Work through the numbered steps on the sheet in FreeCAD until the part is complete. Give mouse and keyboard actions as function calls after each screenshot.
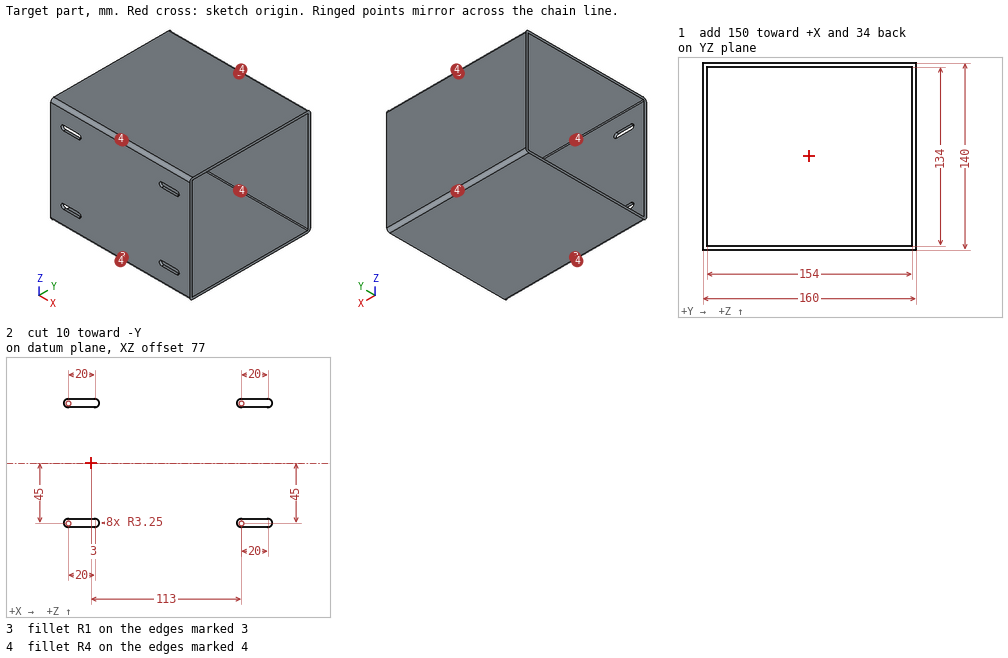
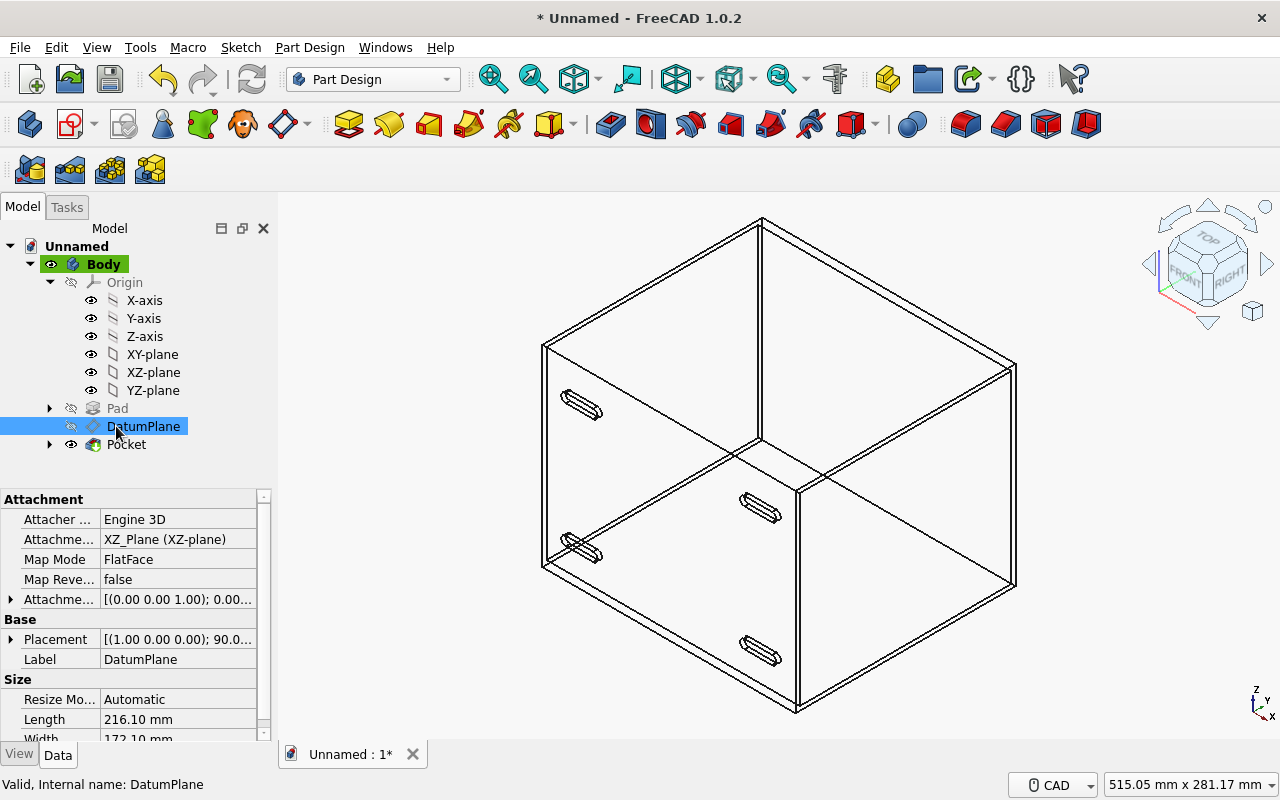
click(885, 297)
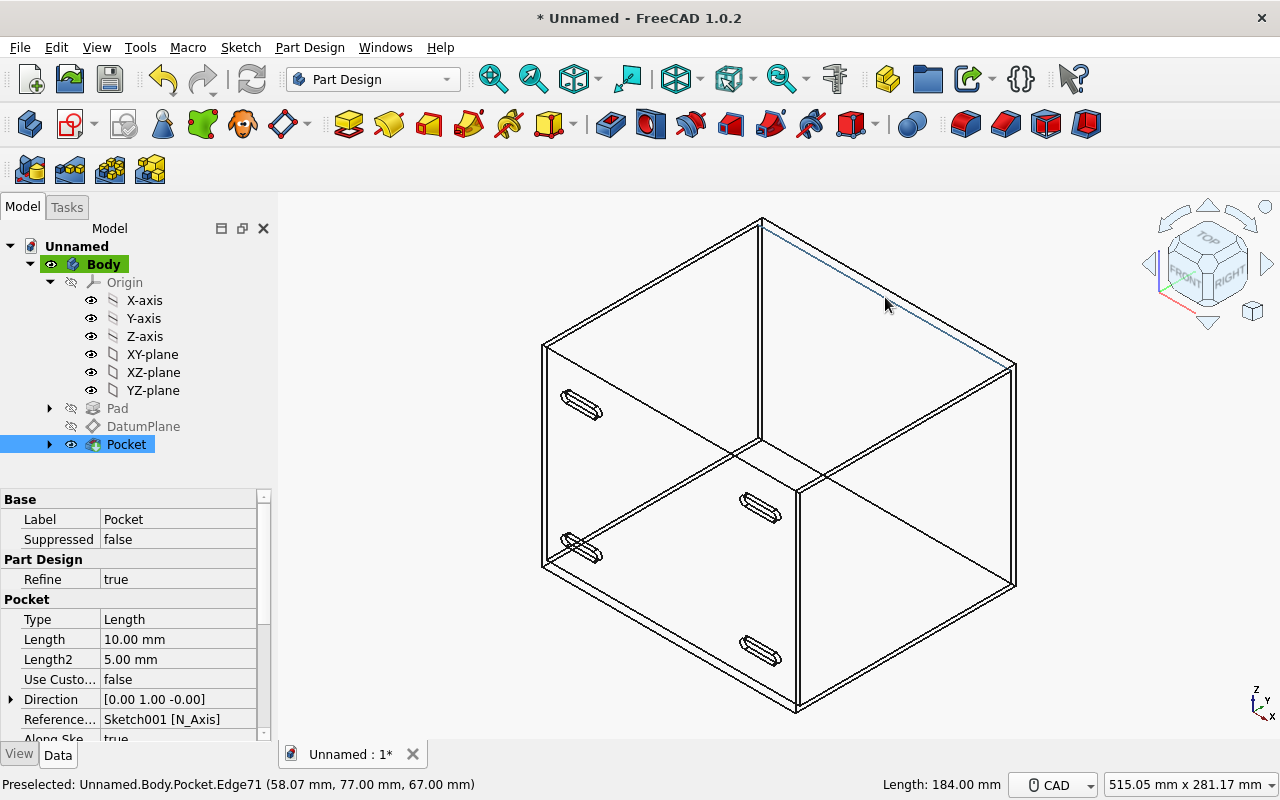
click(885, 510, ctrl)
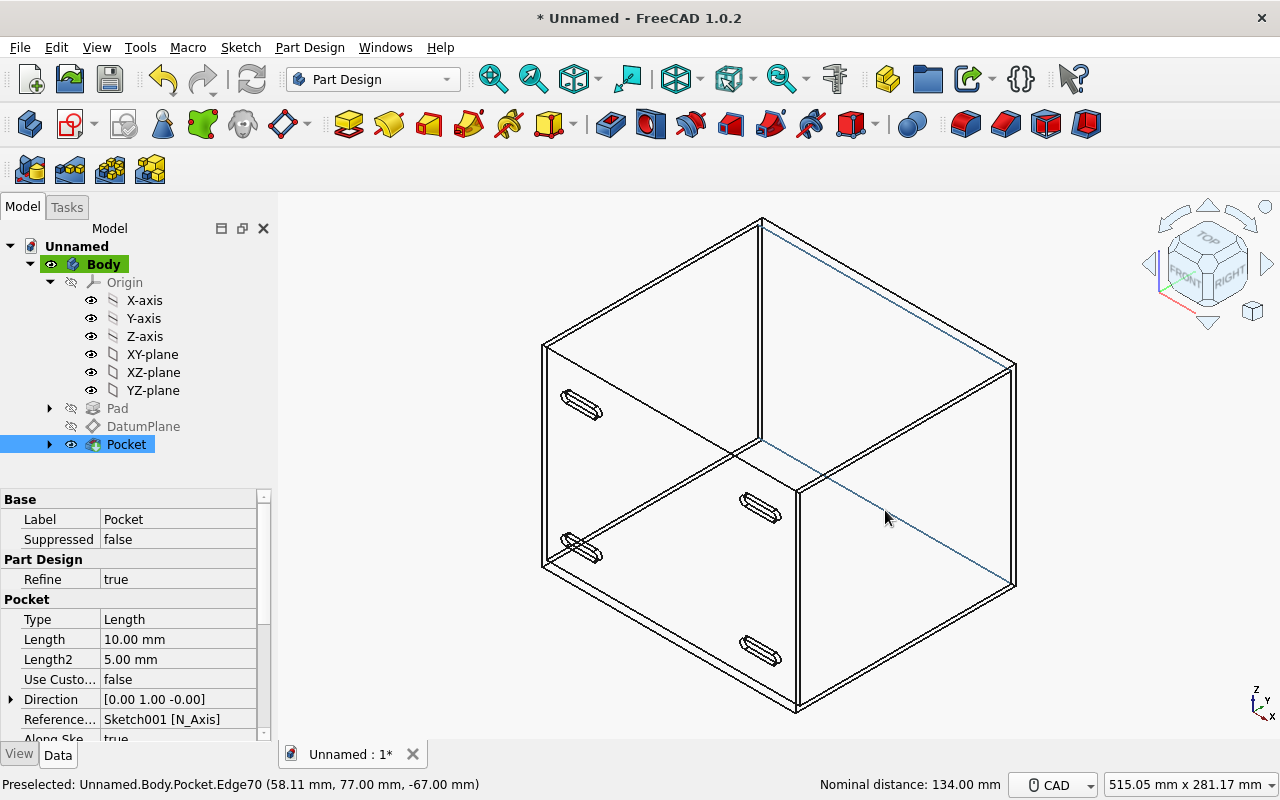
click(673, 632, ctrl)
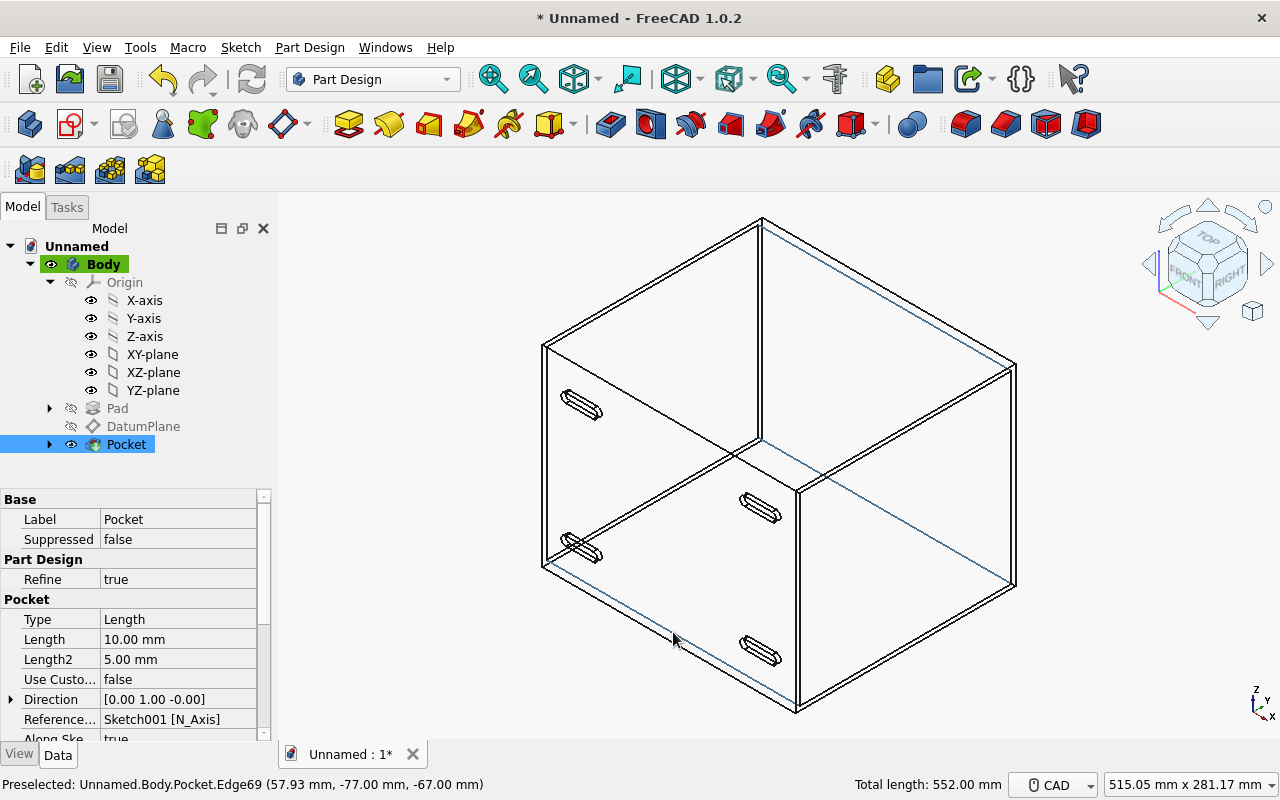
key(2)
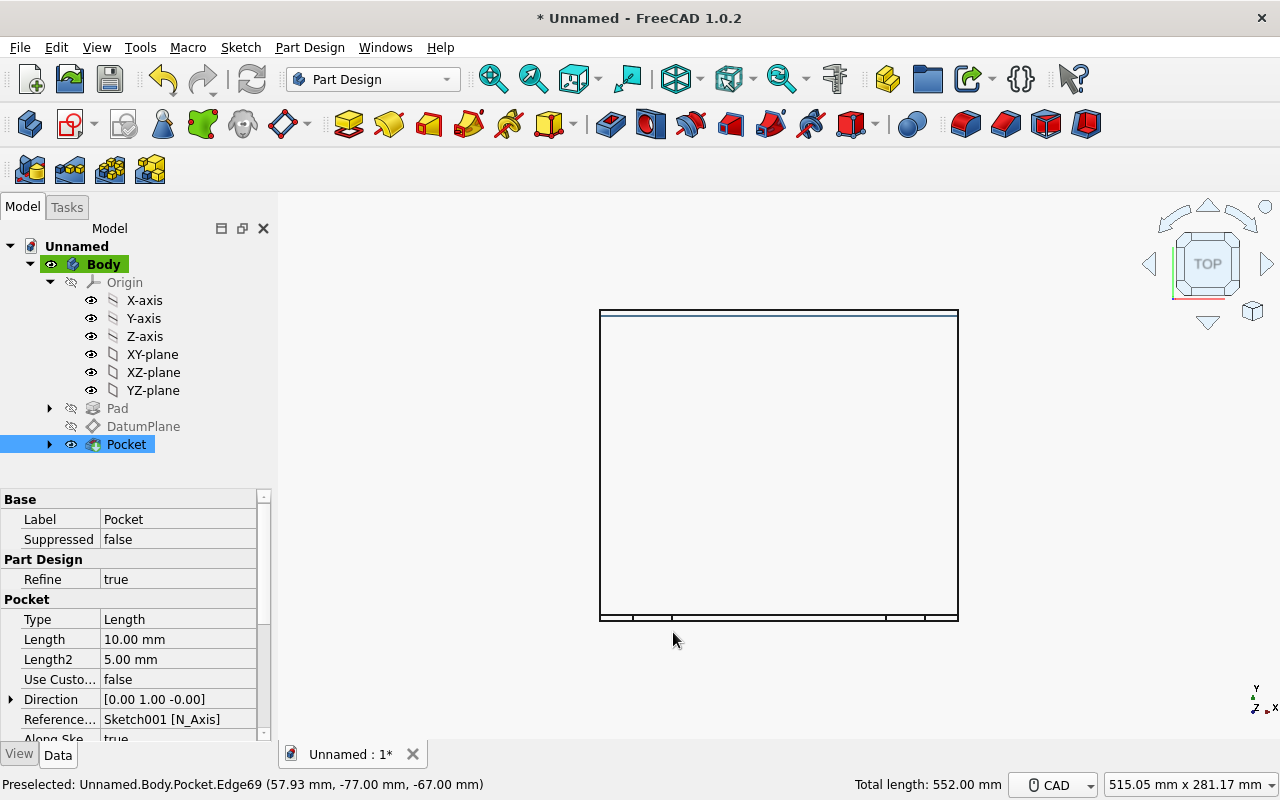
click(779, 614, ctrl)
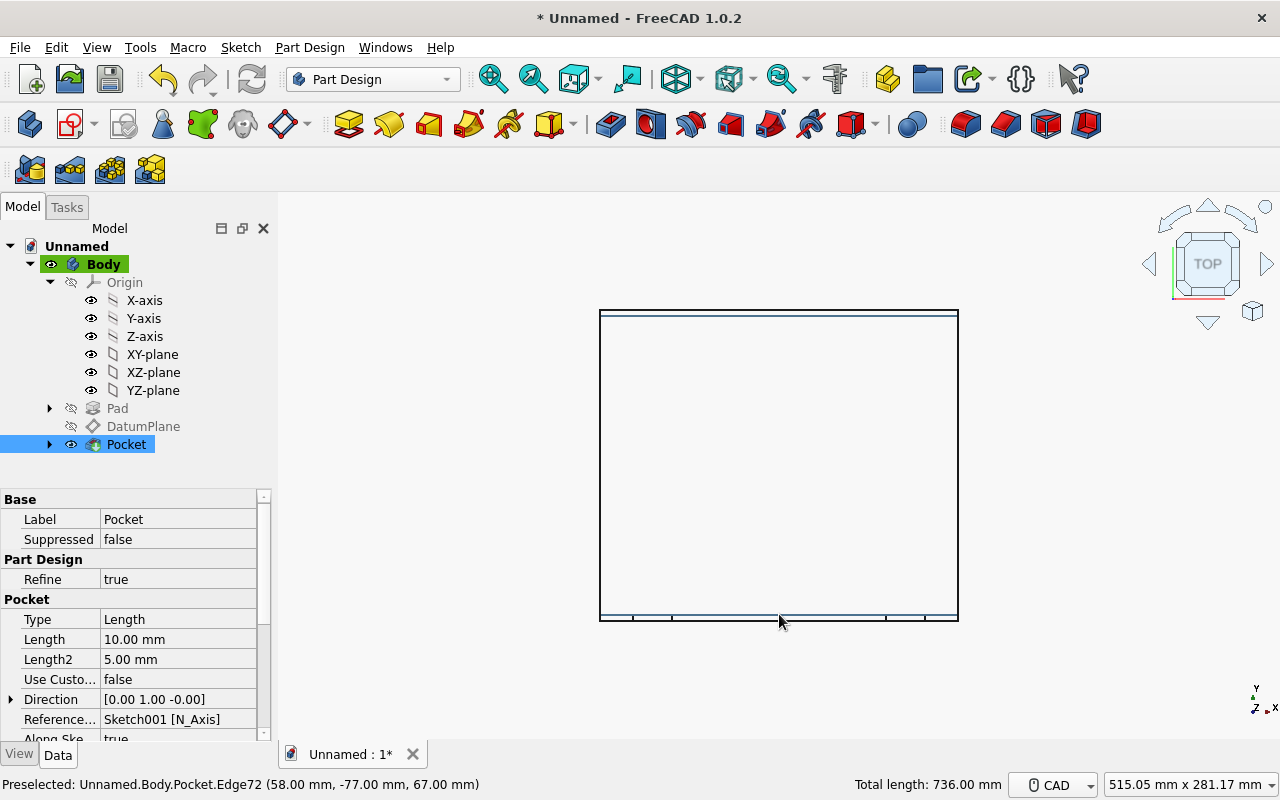
key(v)
key(1)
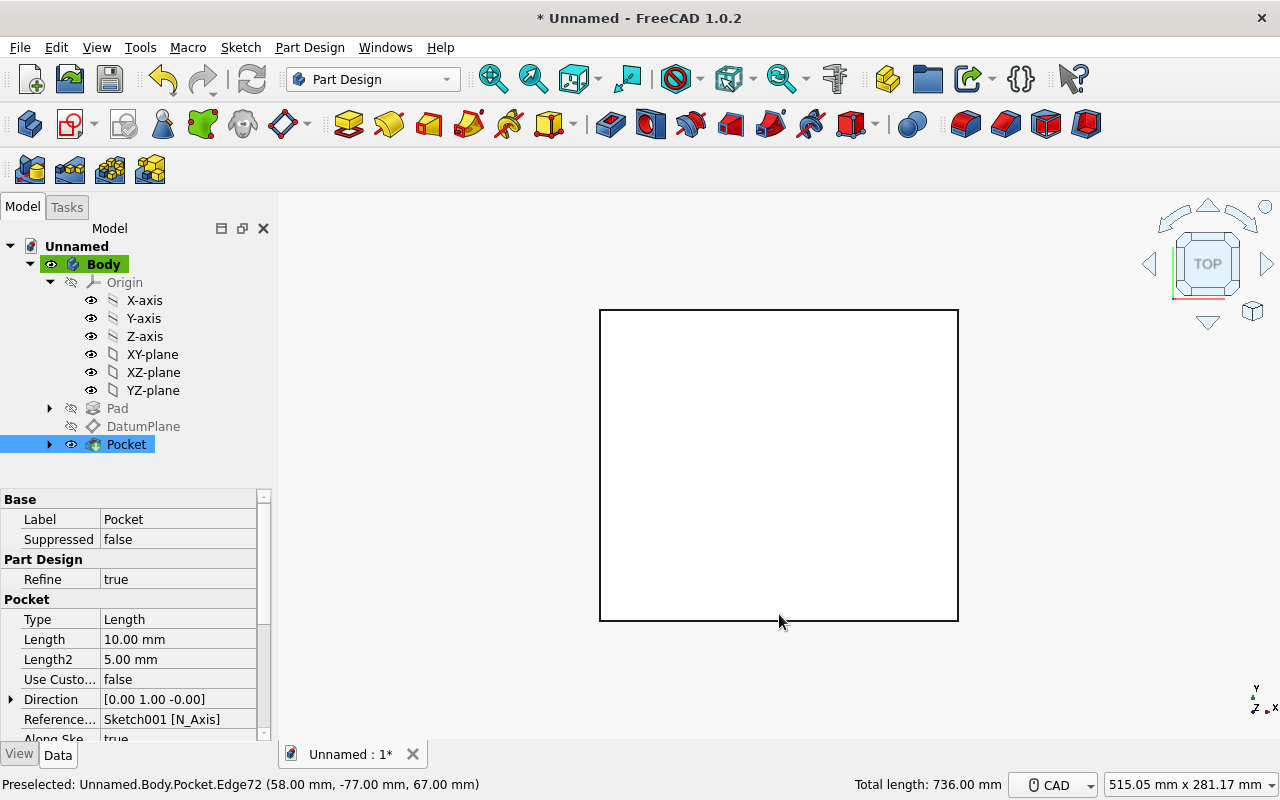
click(966, 124)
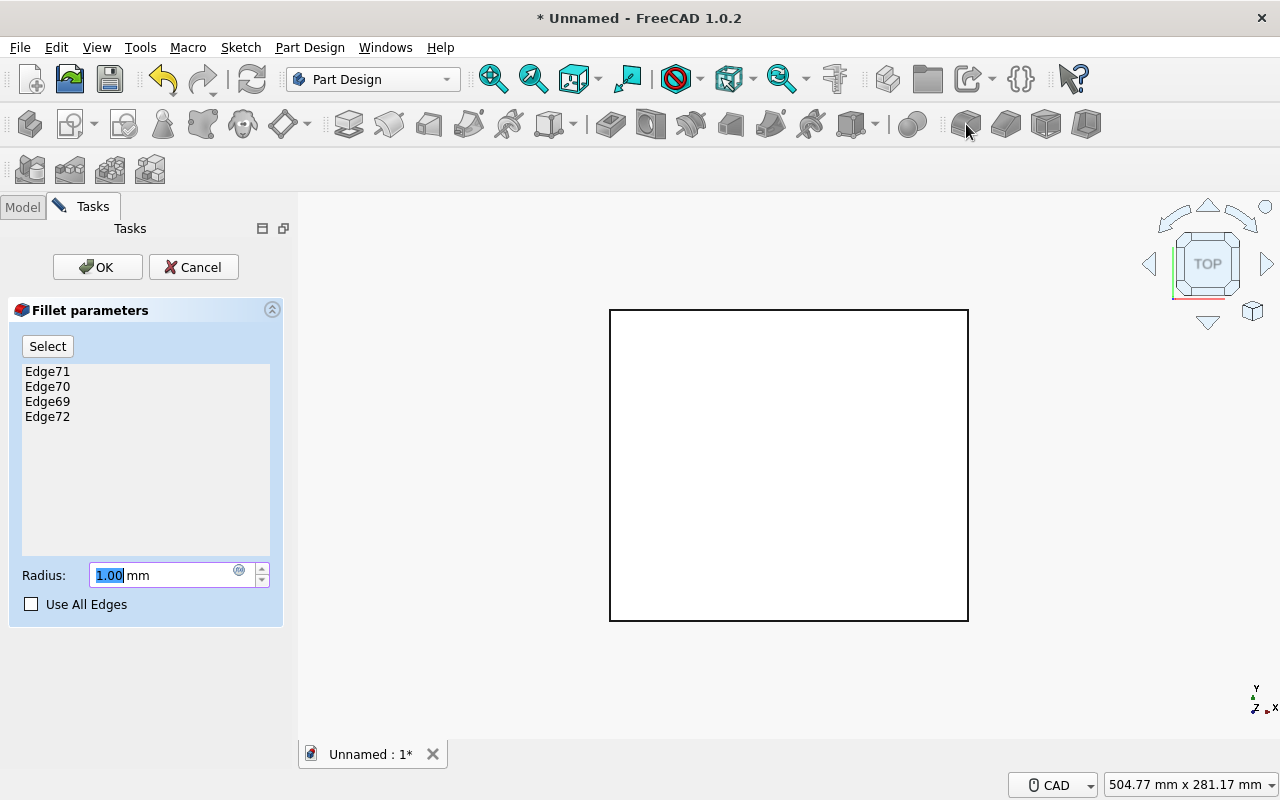
text(1)
key(Tab)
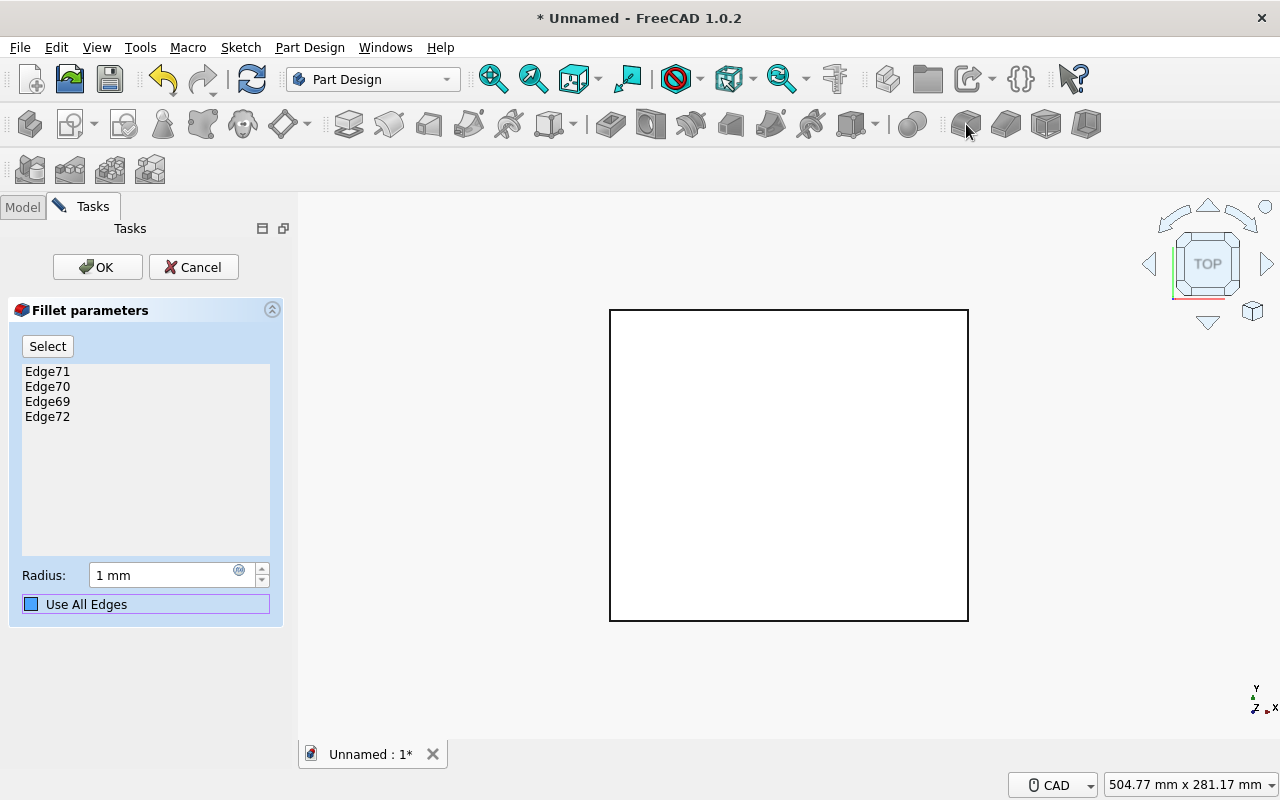
click(98, 267)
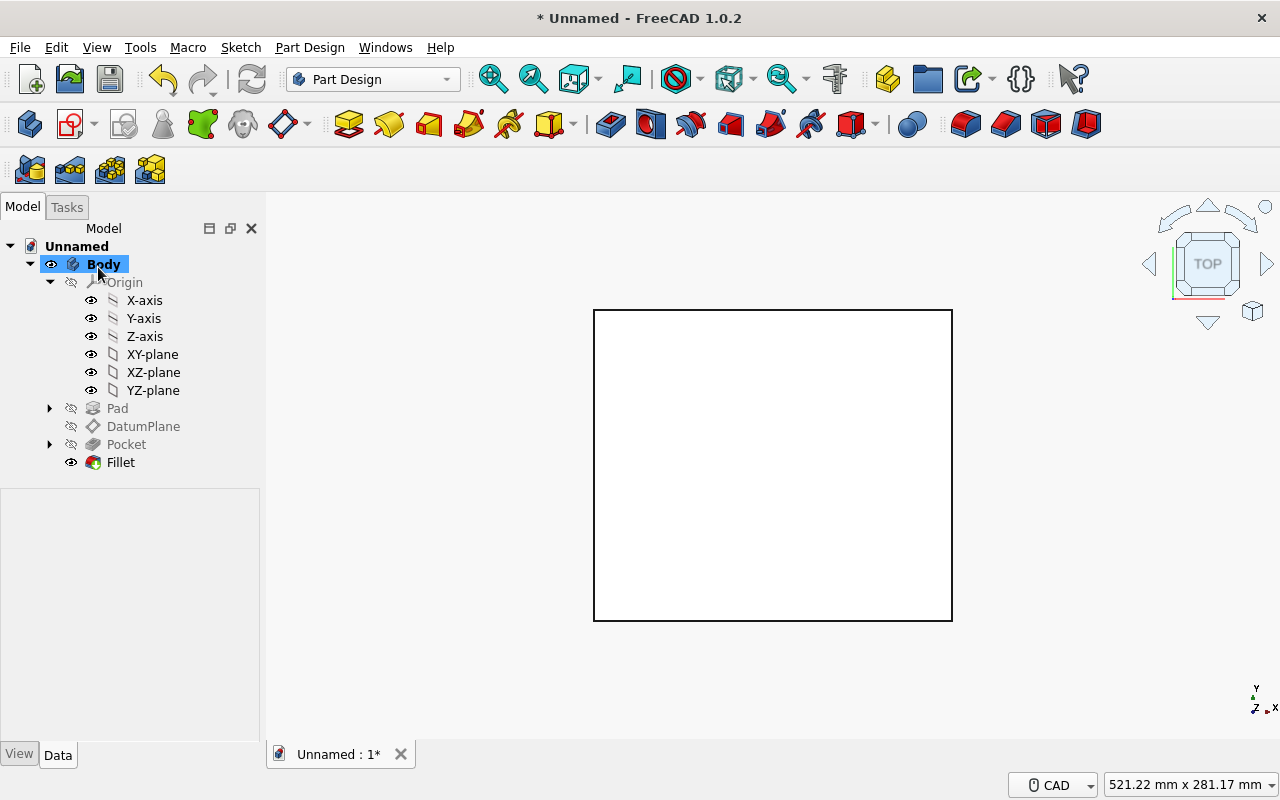
click(773, 620)